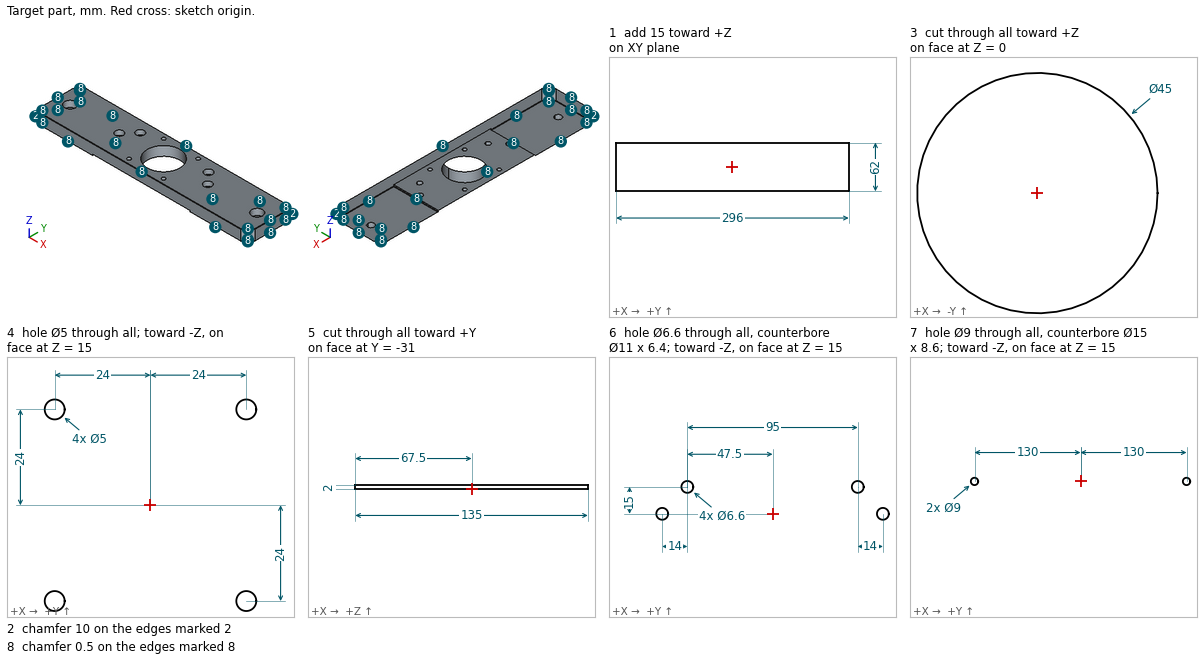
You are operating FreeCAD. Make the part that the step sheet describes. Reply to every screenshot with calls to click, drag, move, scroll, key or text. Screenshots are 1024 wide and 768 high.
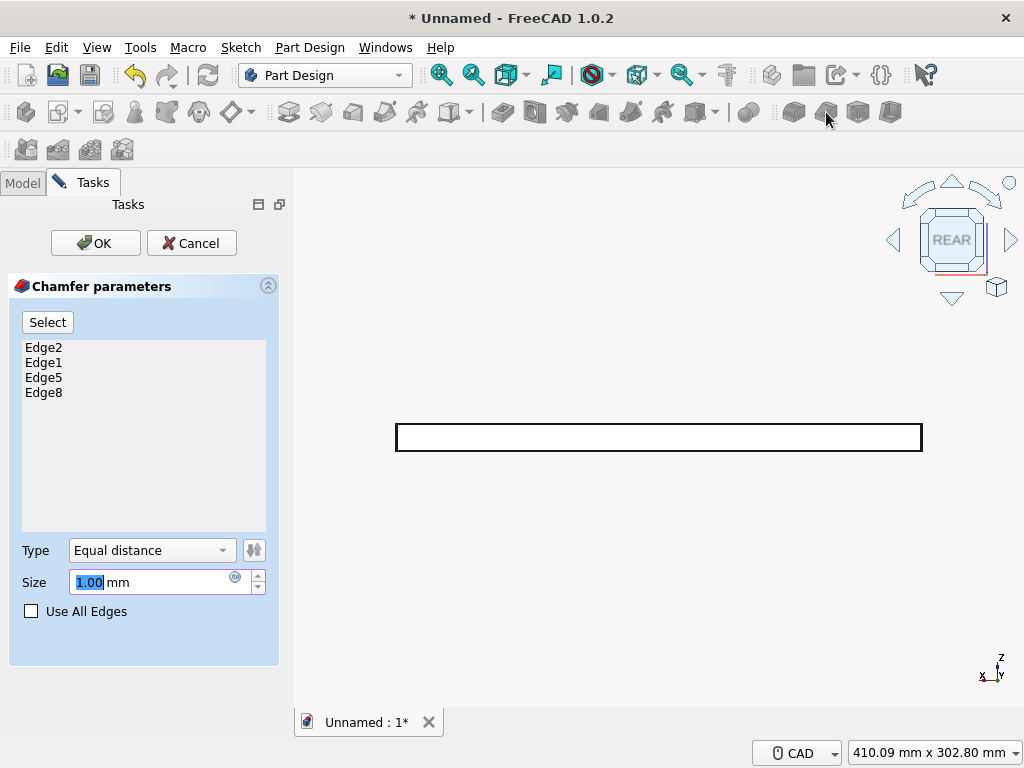
text(10)
key(Tab)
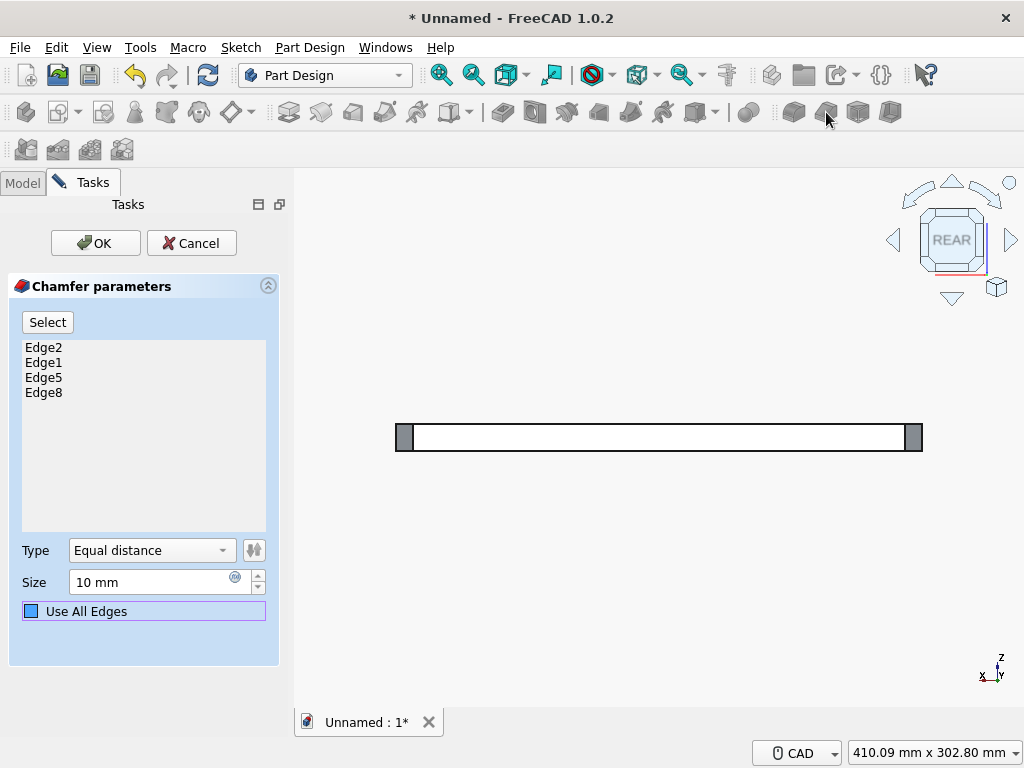
click(96, 243)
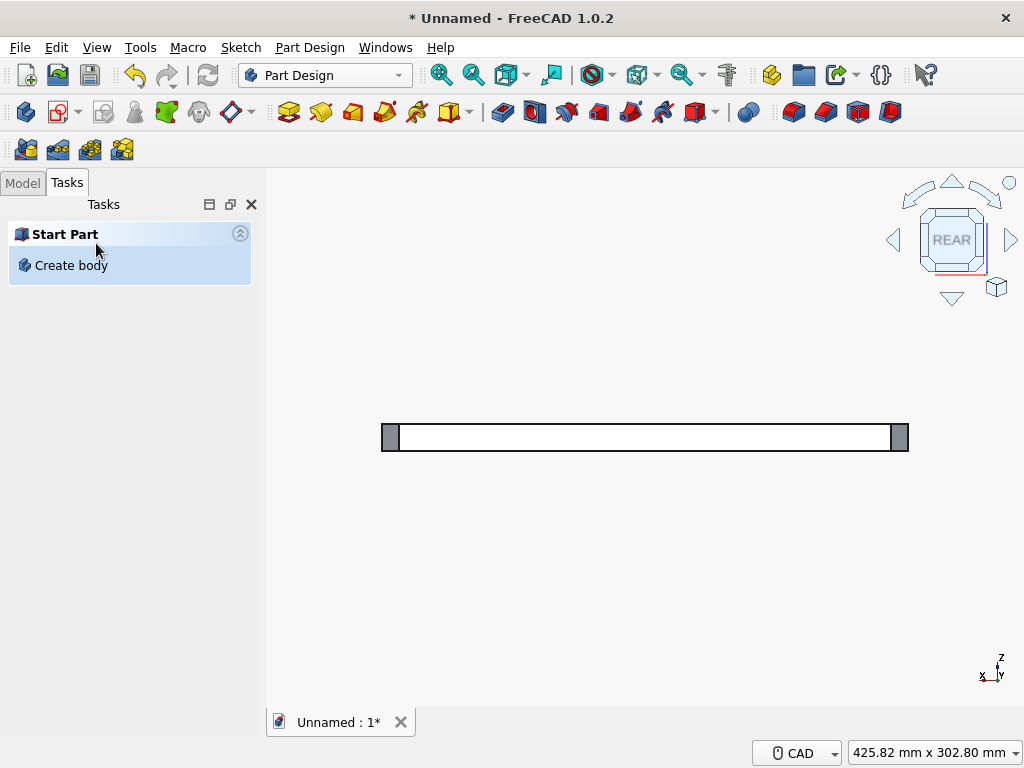
key(5)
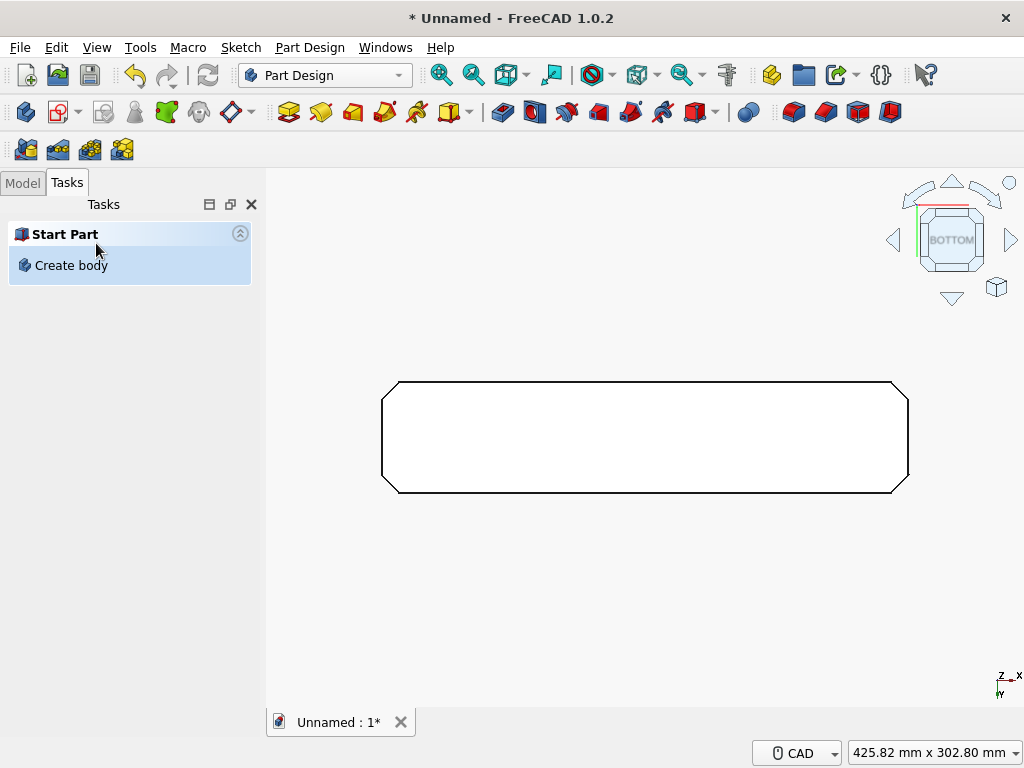
click(796, 436)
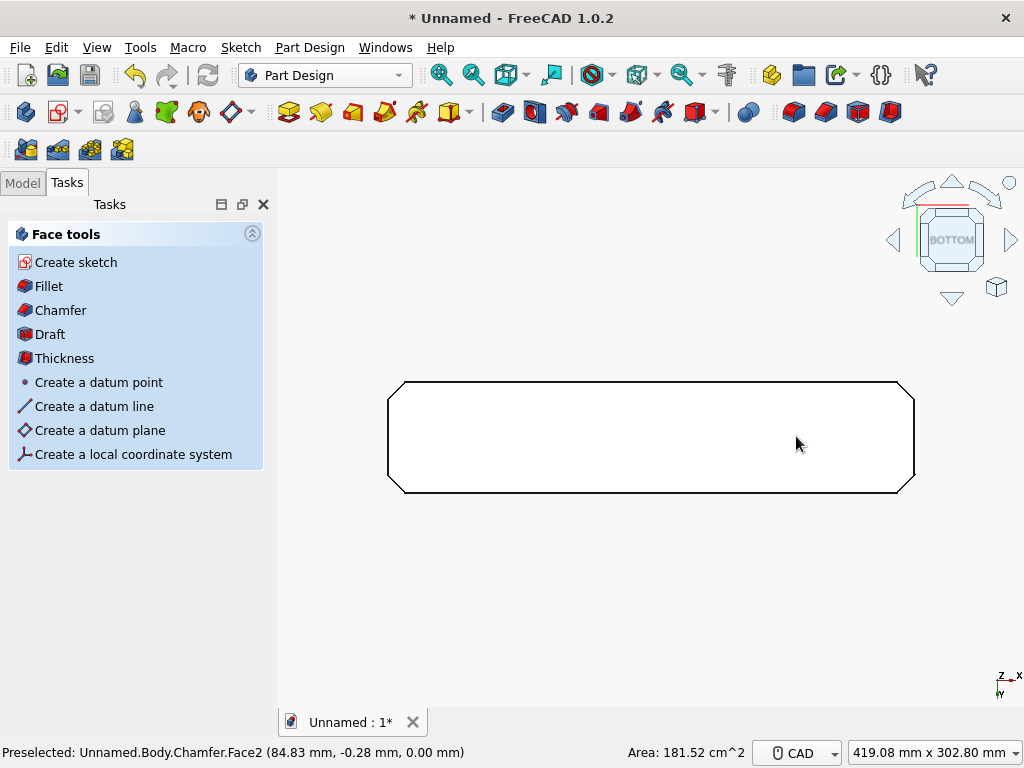
click(58, 112)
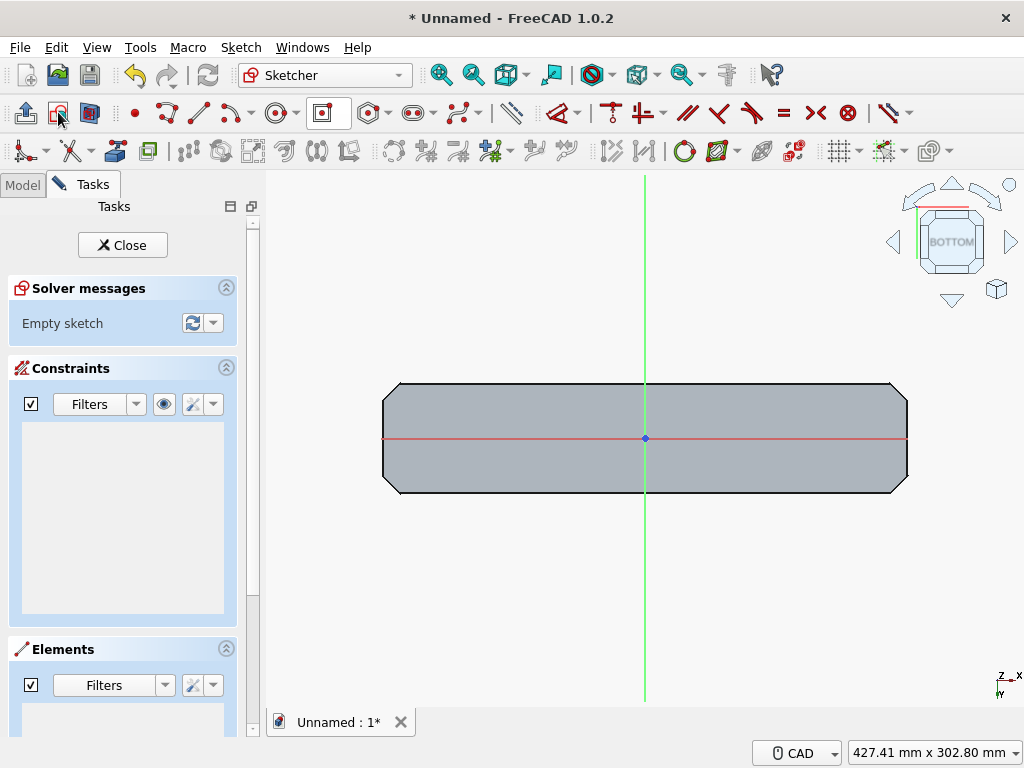
scroll(667, 438, up, 7)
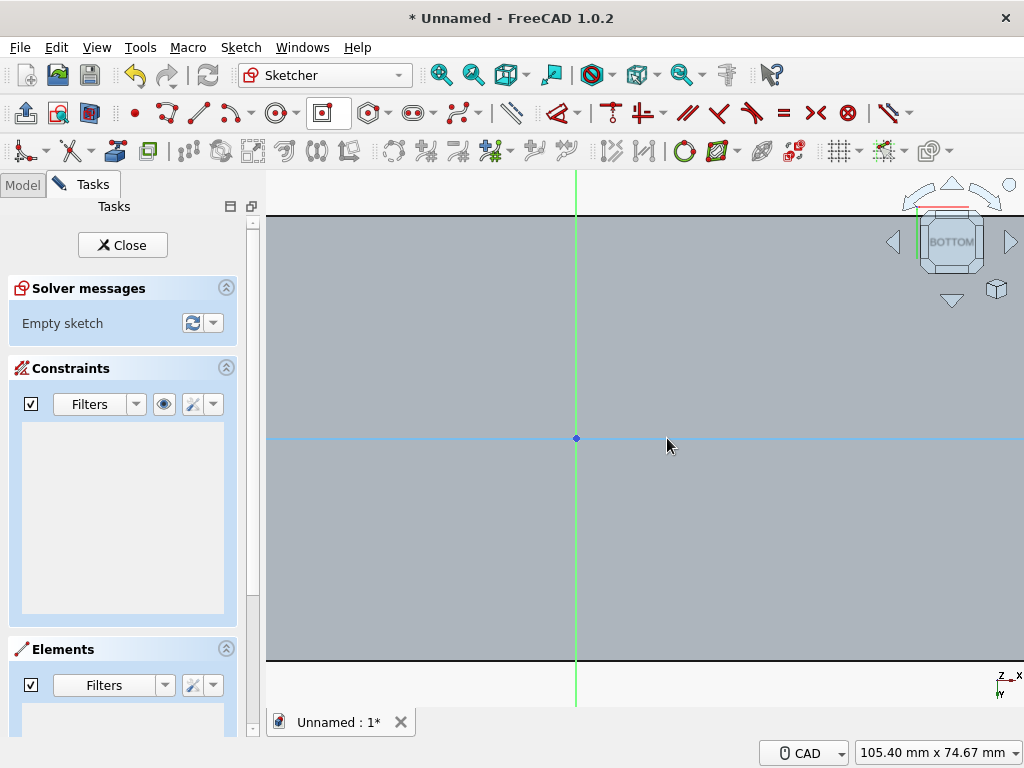
click(276, 114)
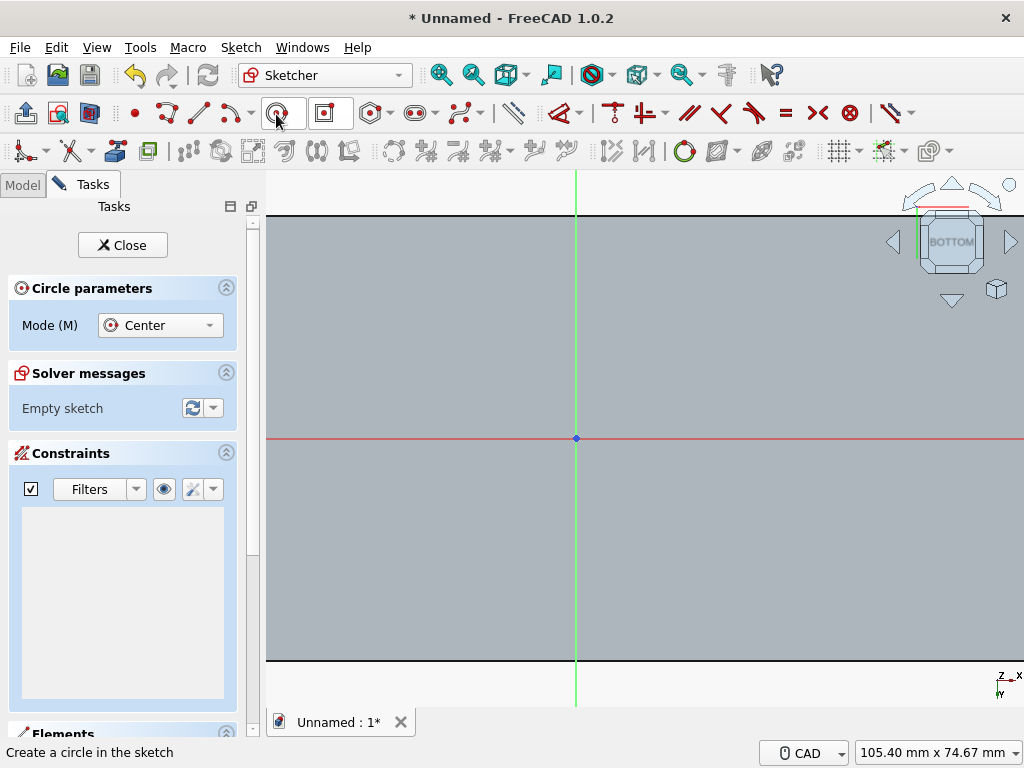
click(576, 438)
move(691, 324)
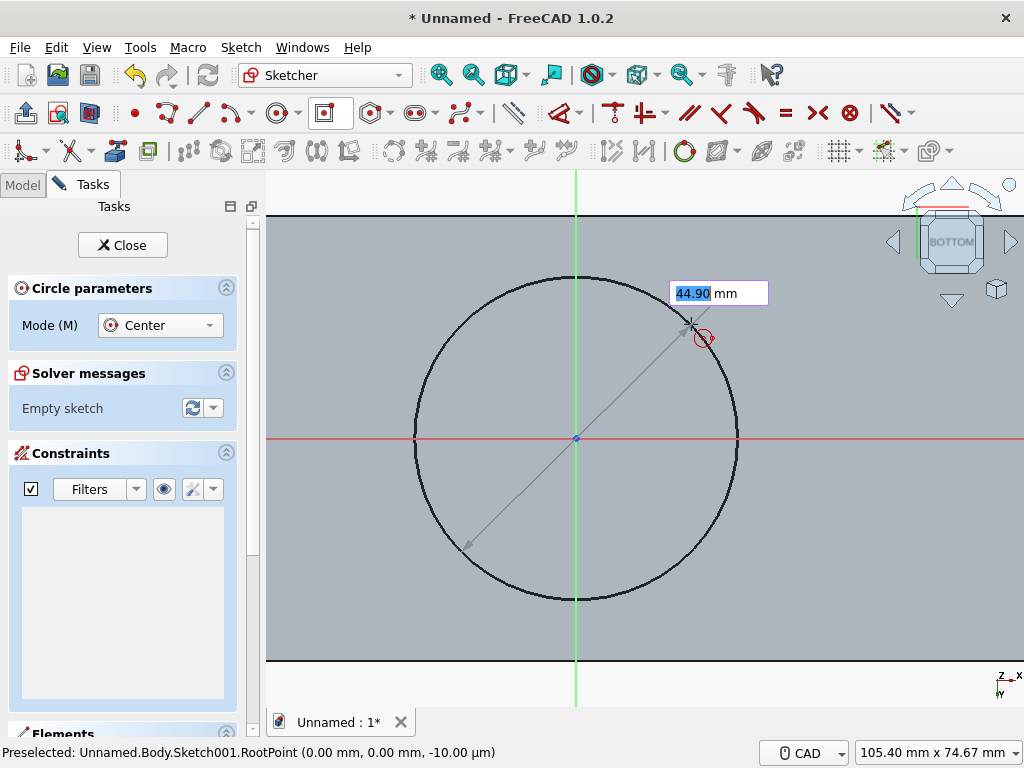
text(45)
key(Return)
key(Escape)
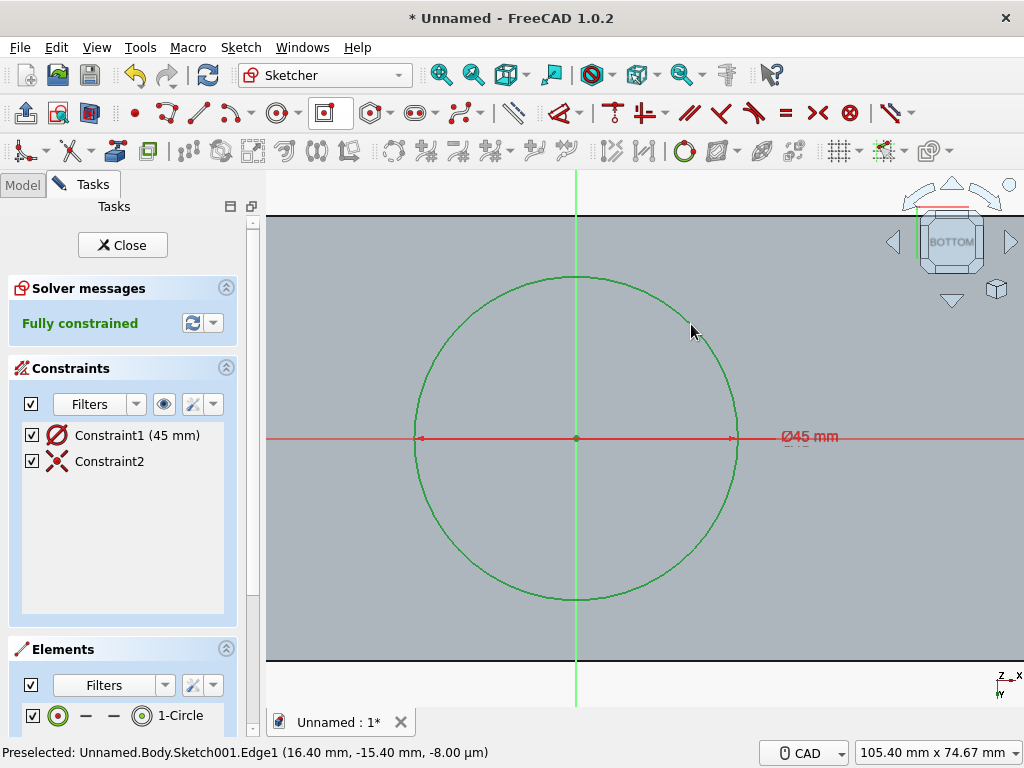
click(123, 245)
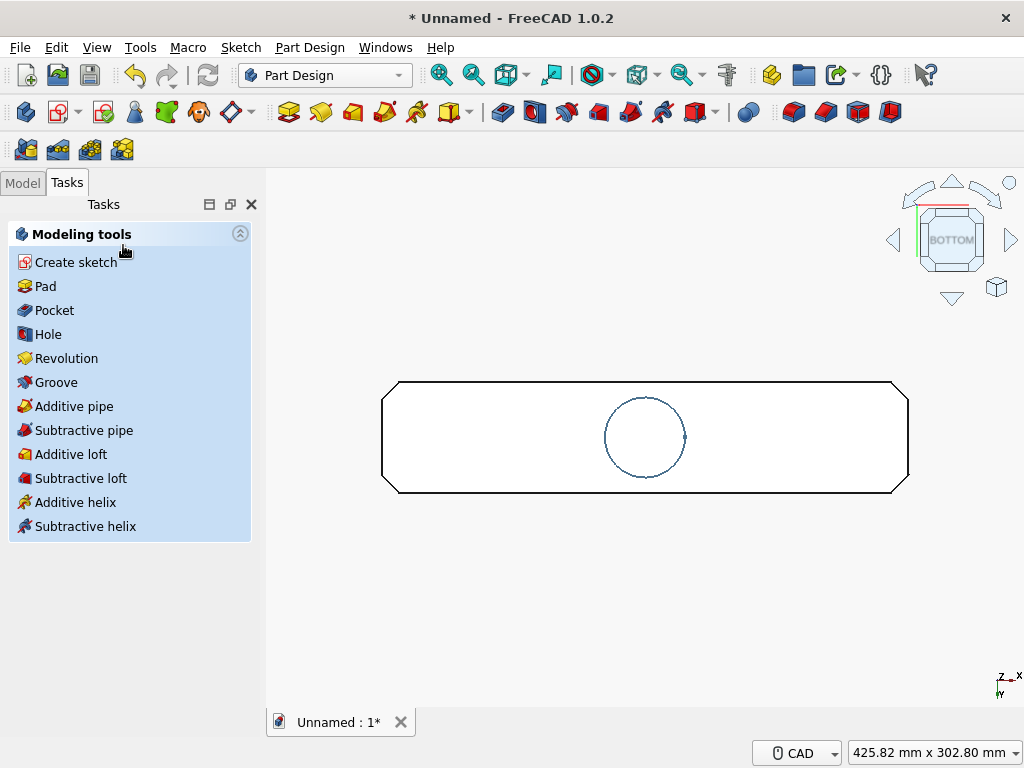
click(504, 112)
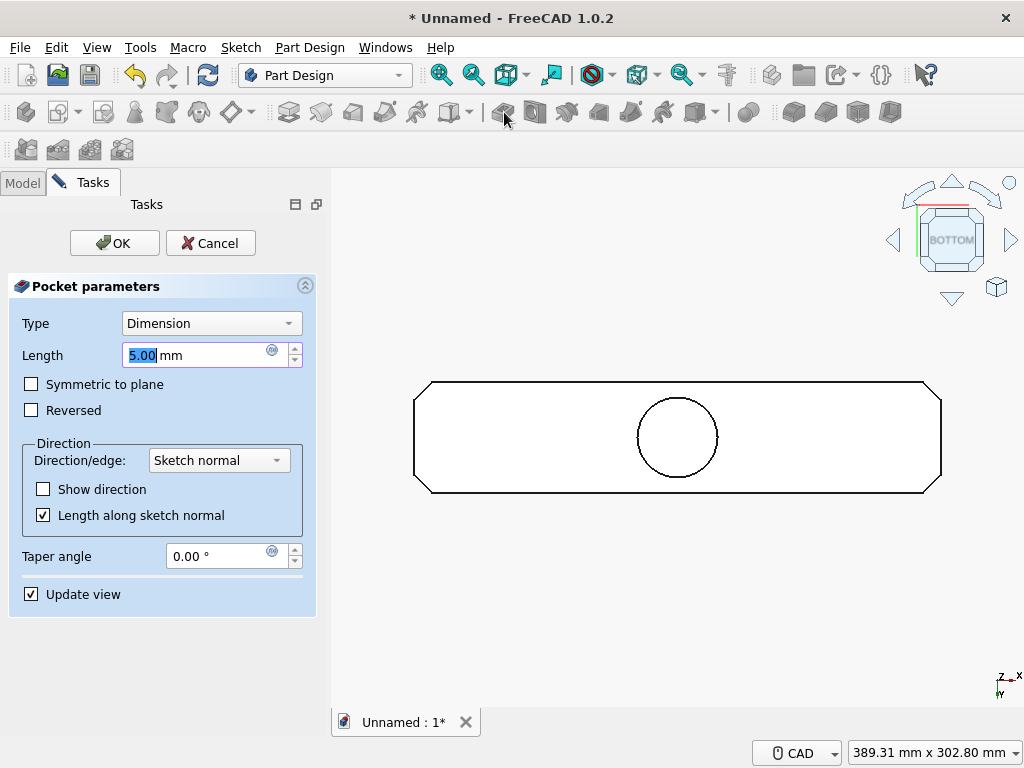
click(212, 324)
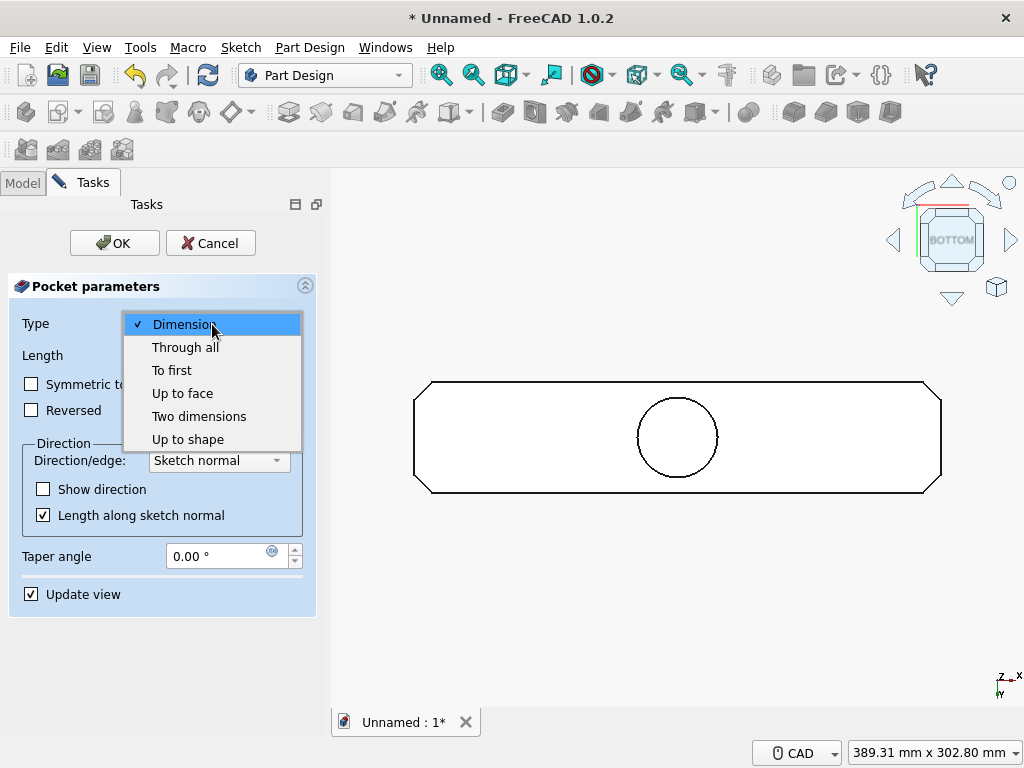
click(212, 348)